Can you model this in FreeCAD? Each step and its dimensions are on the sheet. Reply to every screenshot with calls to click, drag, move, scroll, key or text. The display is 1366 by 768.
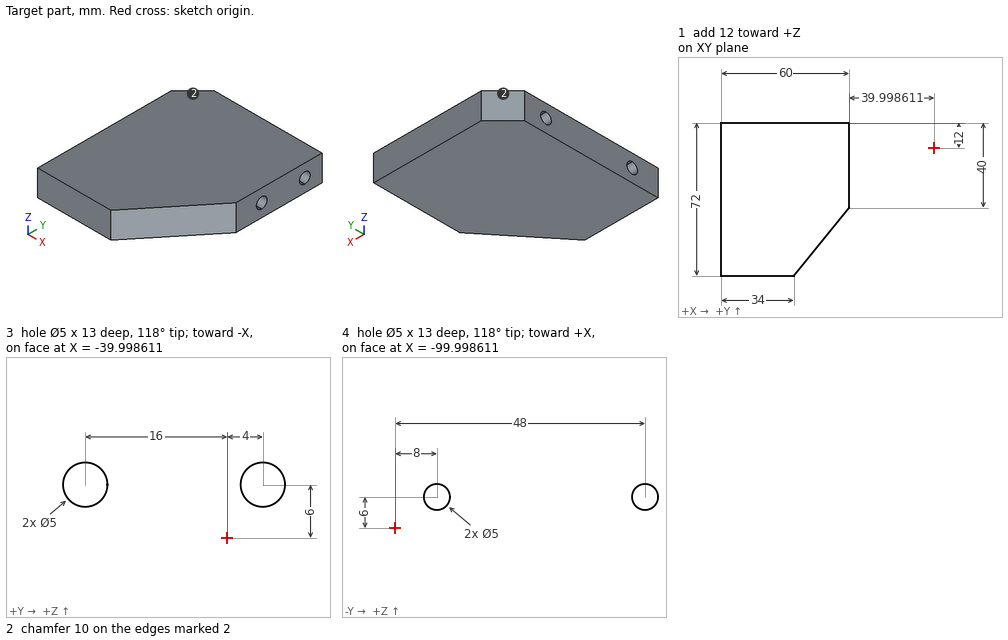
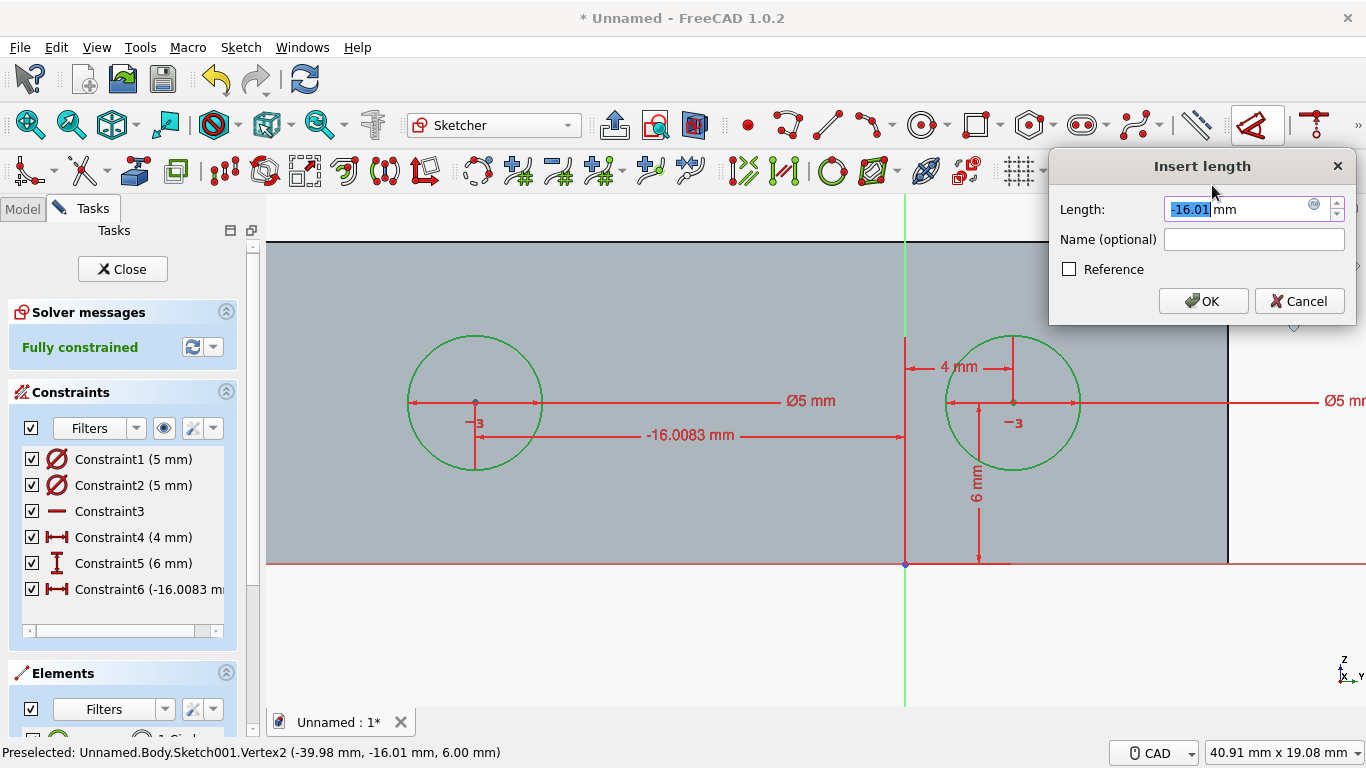
text(-16)
key(Return)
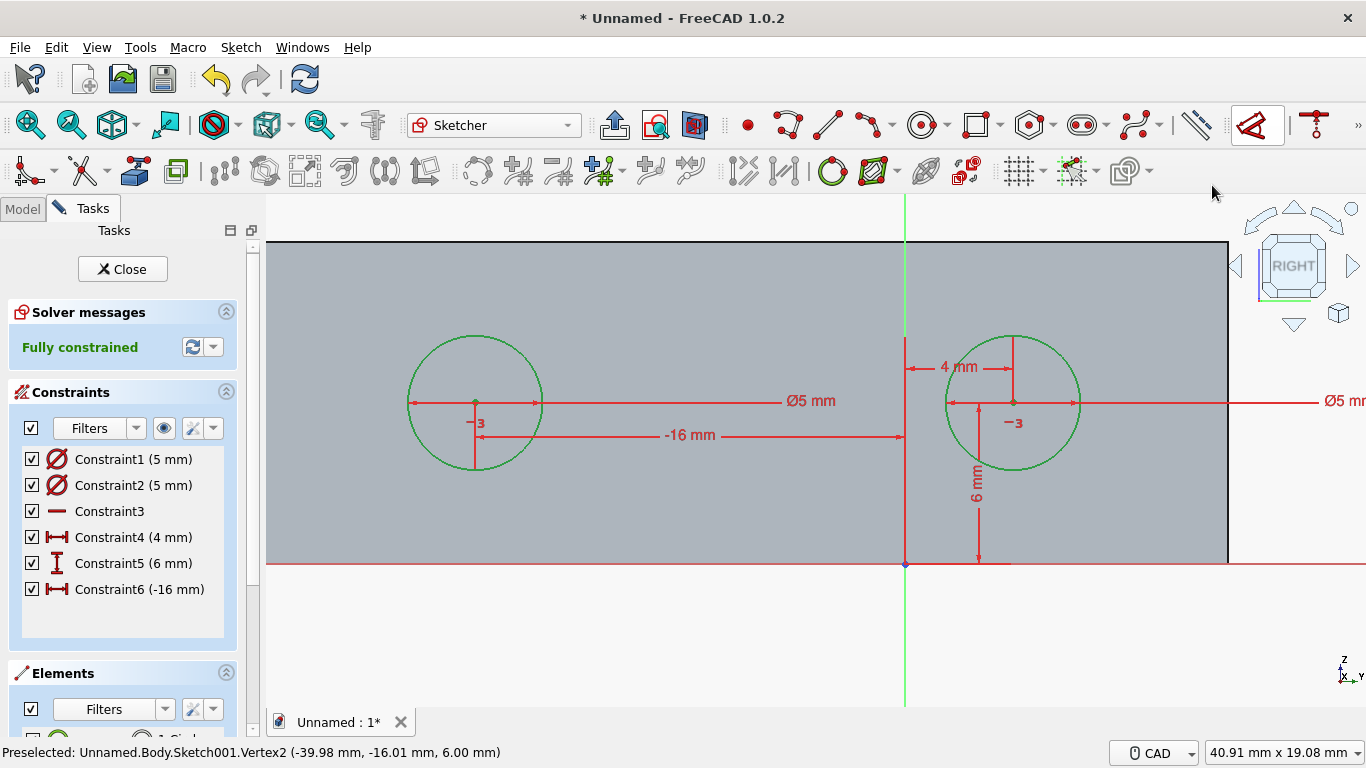
click(123, 269)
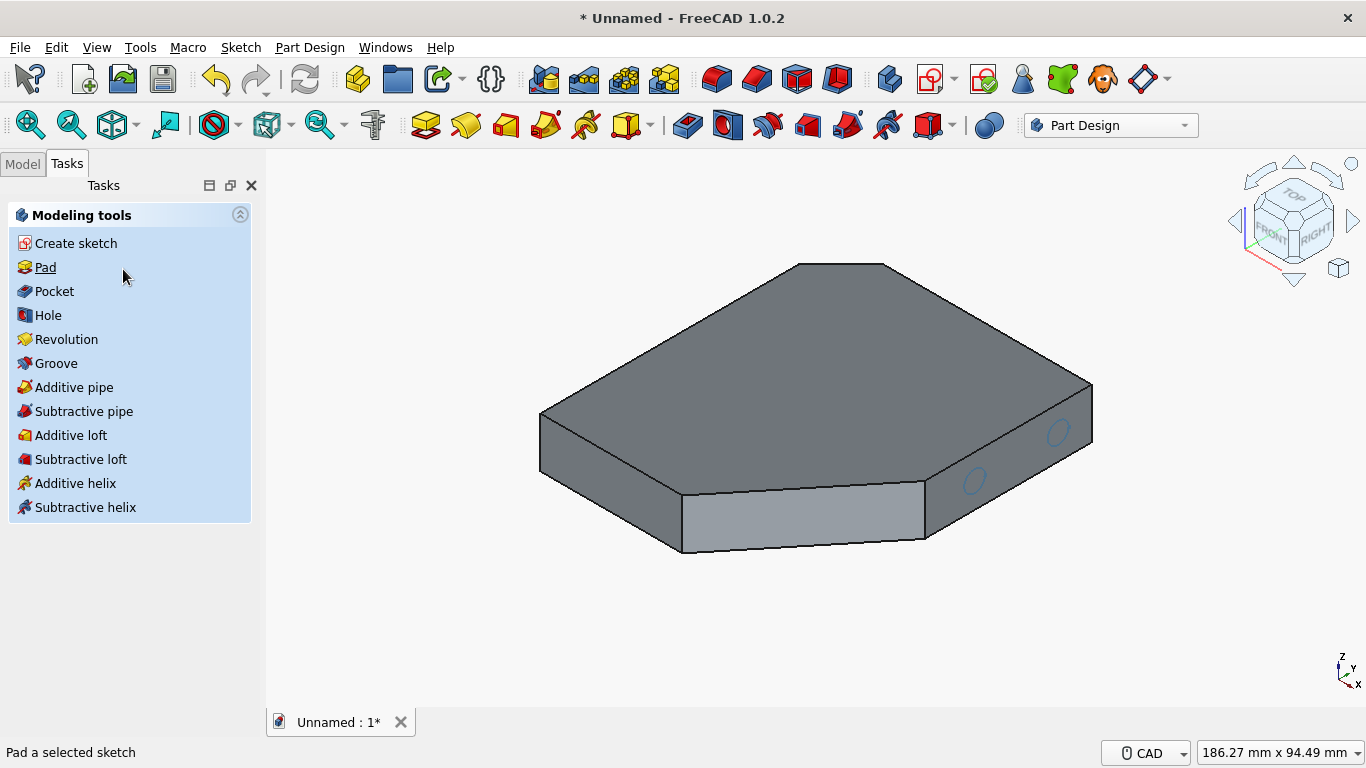
click(728, 126)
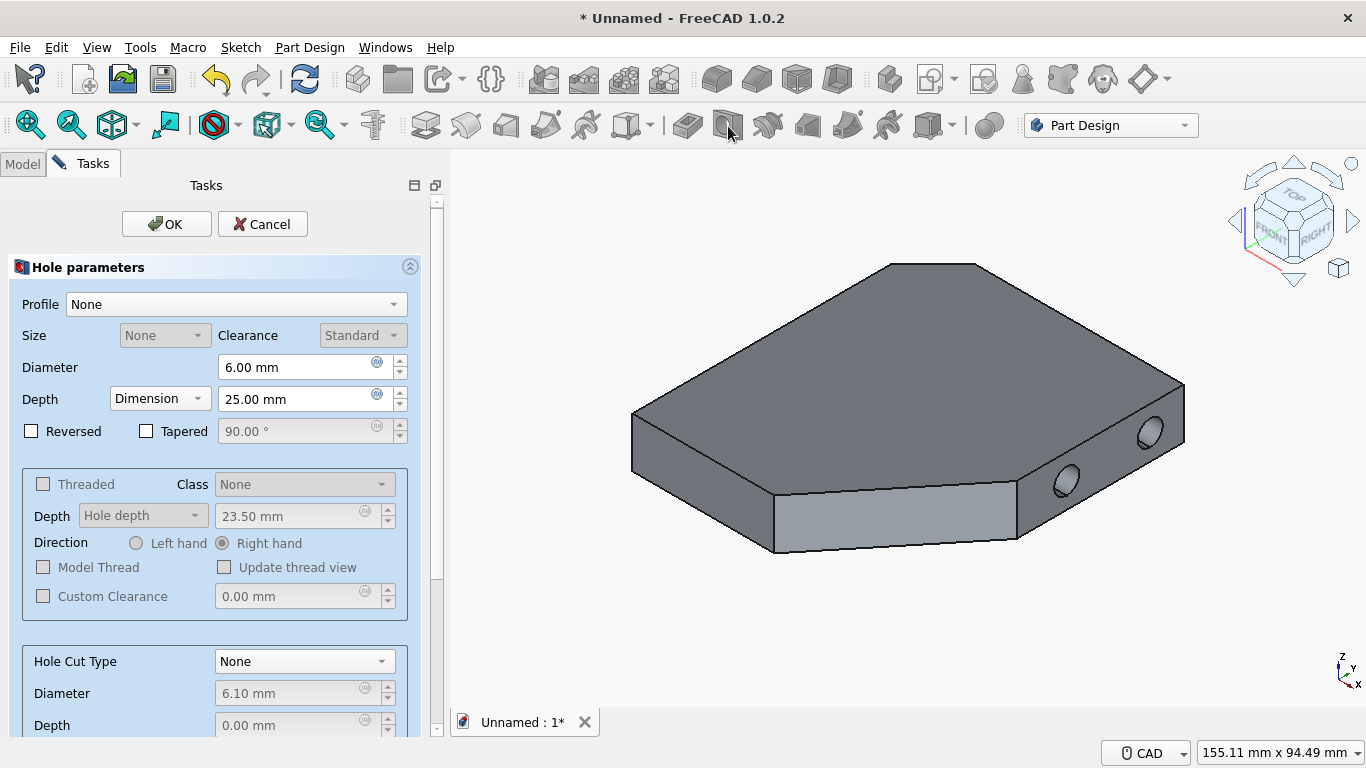
triple_click(305, 367)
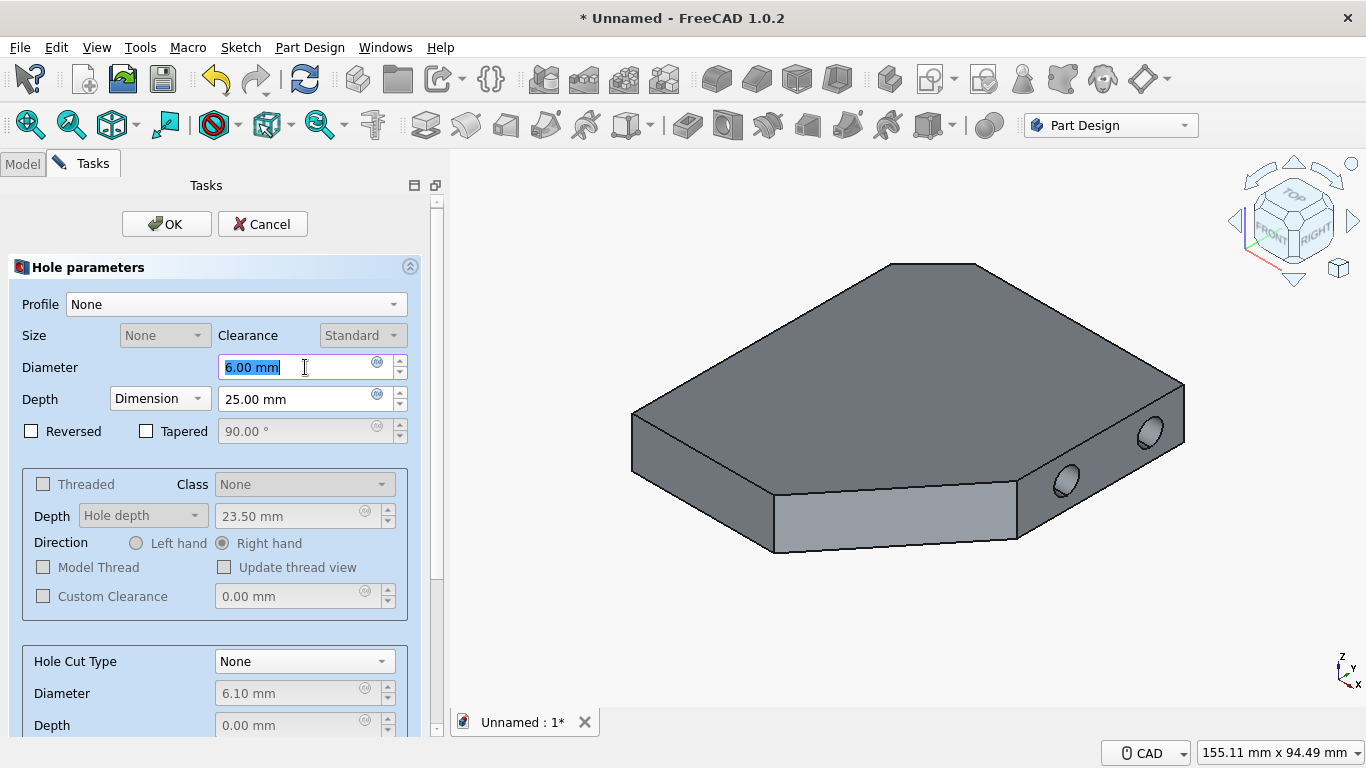
text(5)
key(Tab)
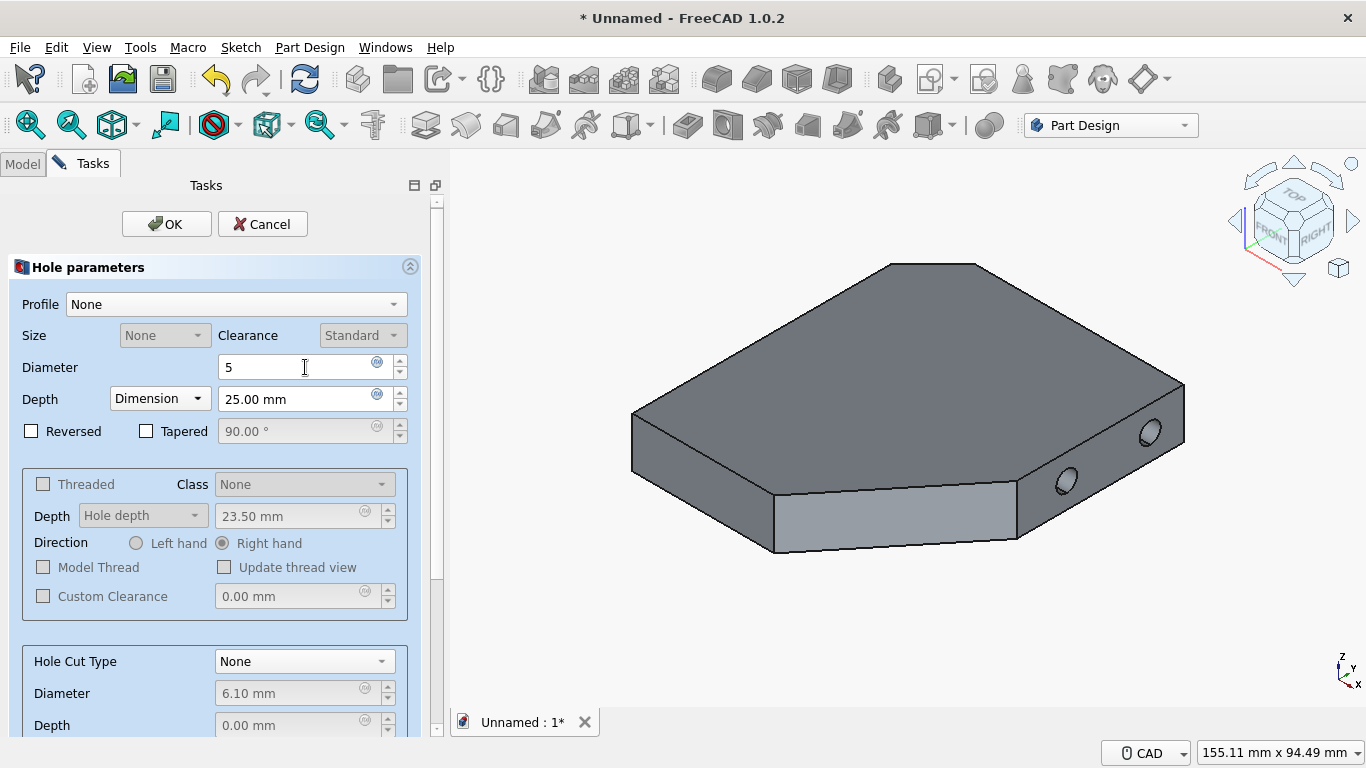
triple_click(305, 399)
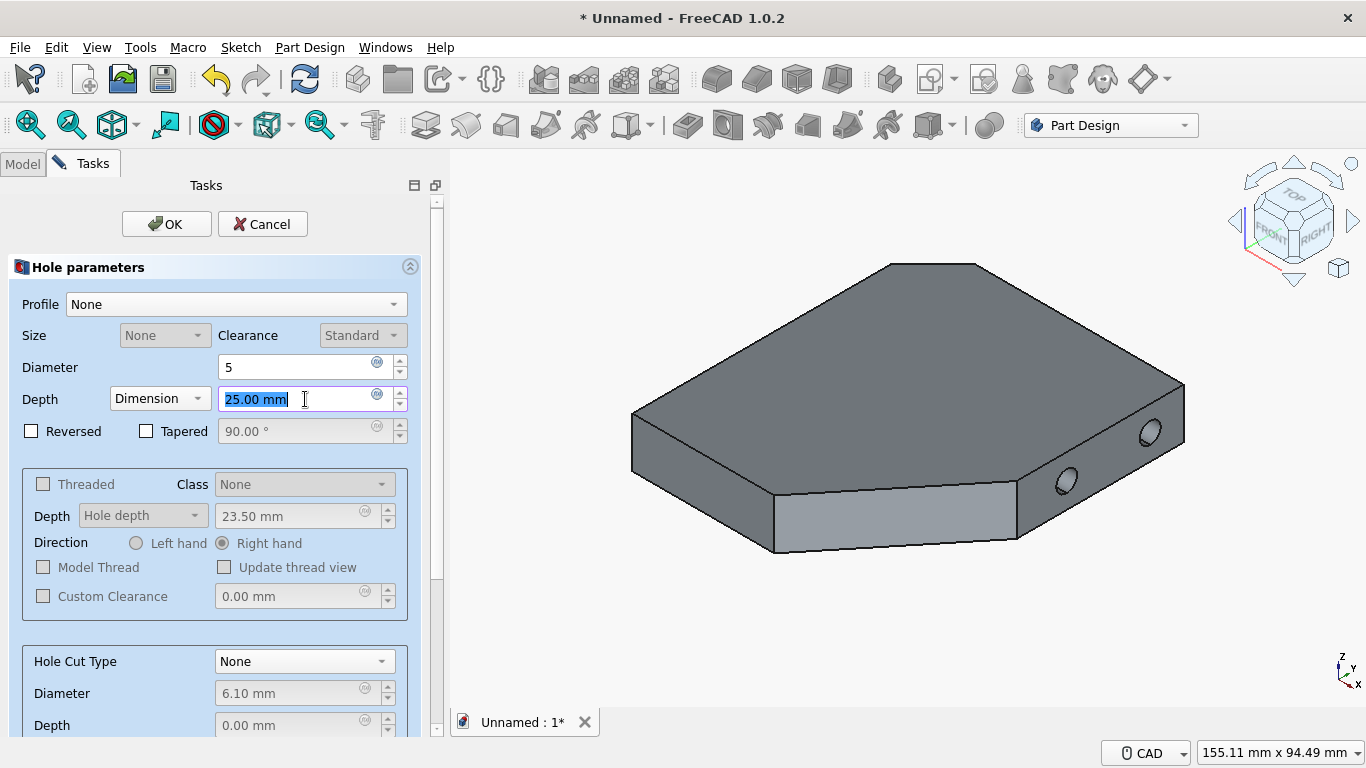
text(13)
key(Tab)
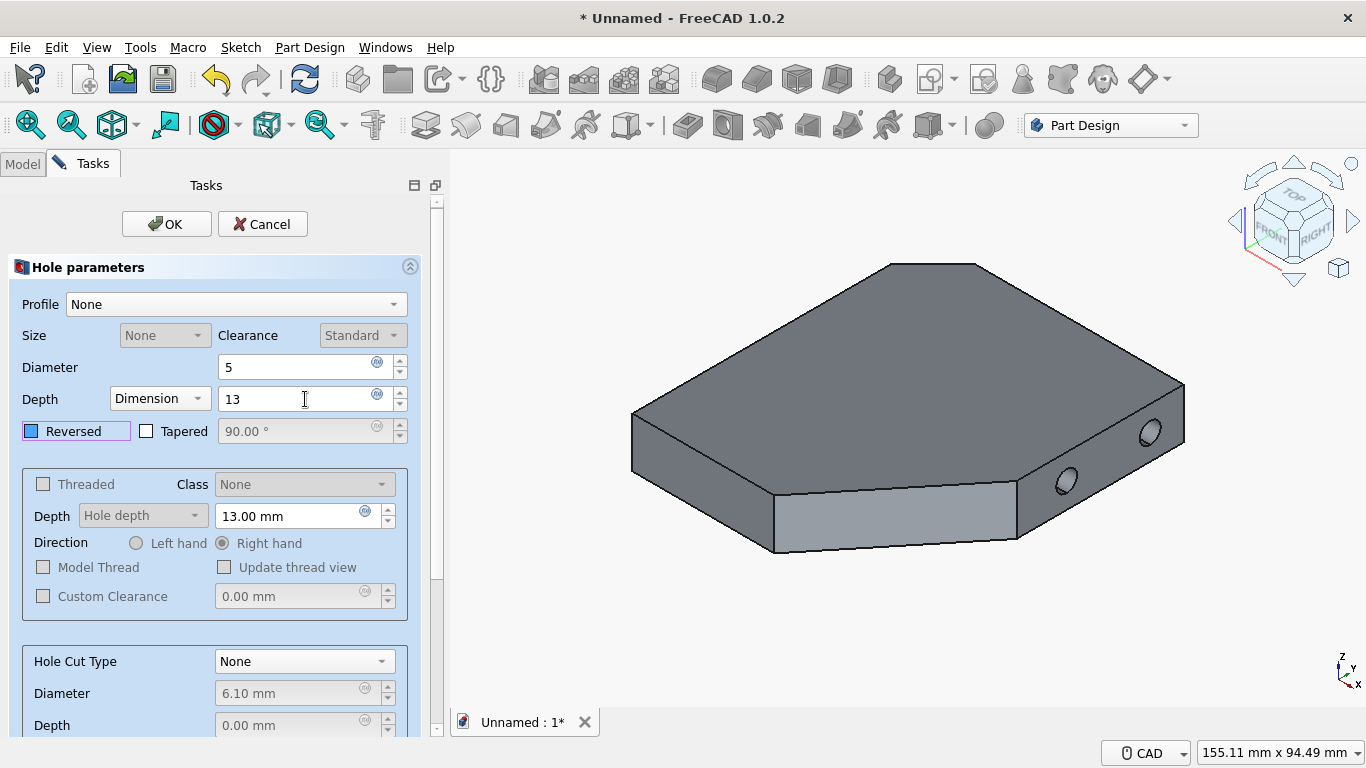
click(167, 224)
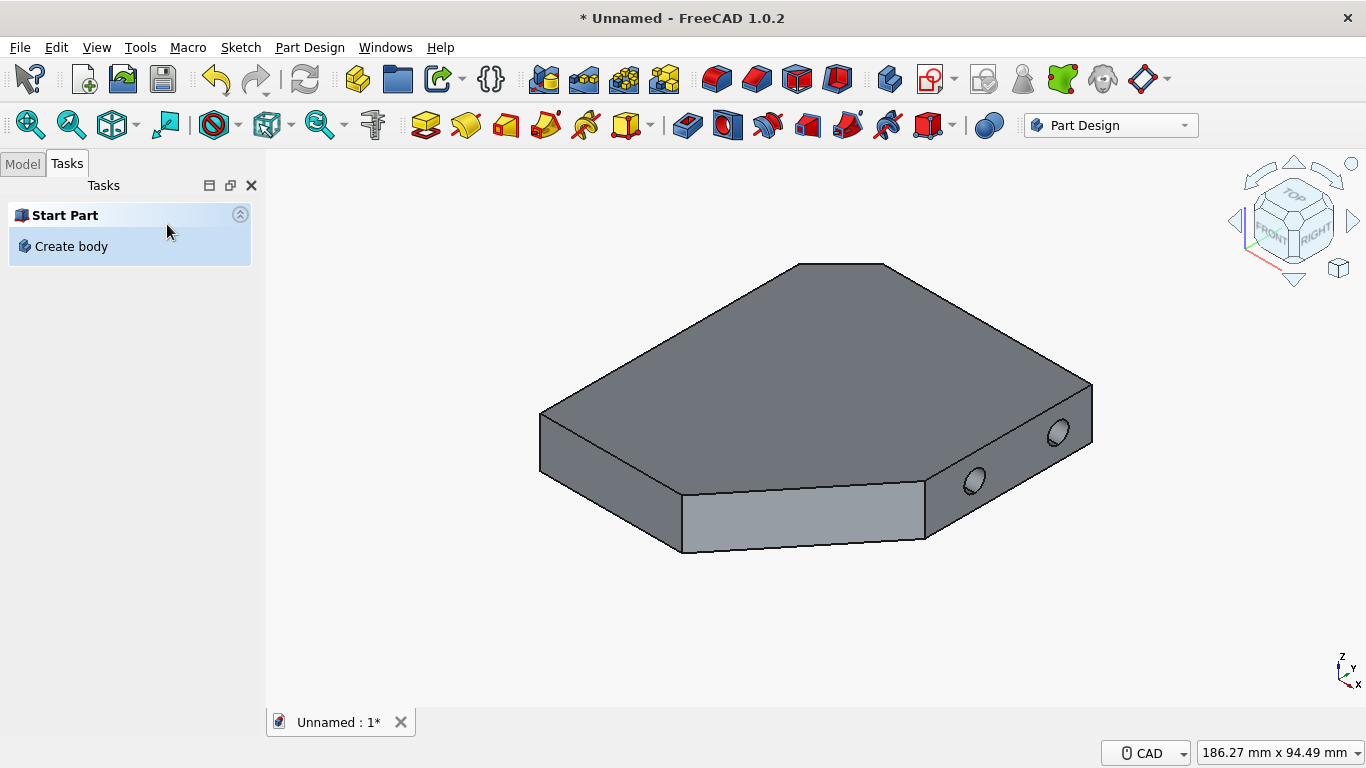
key(6)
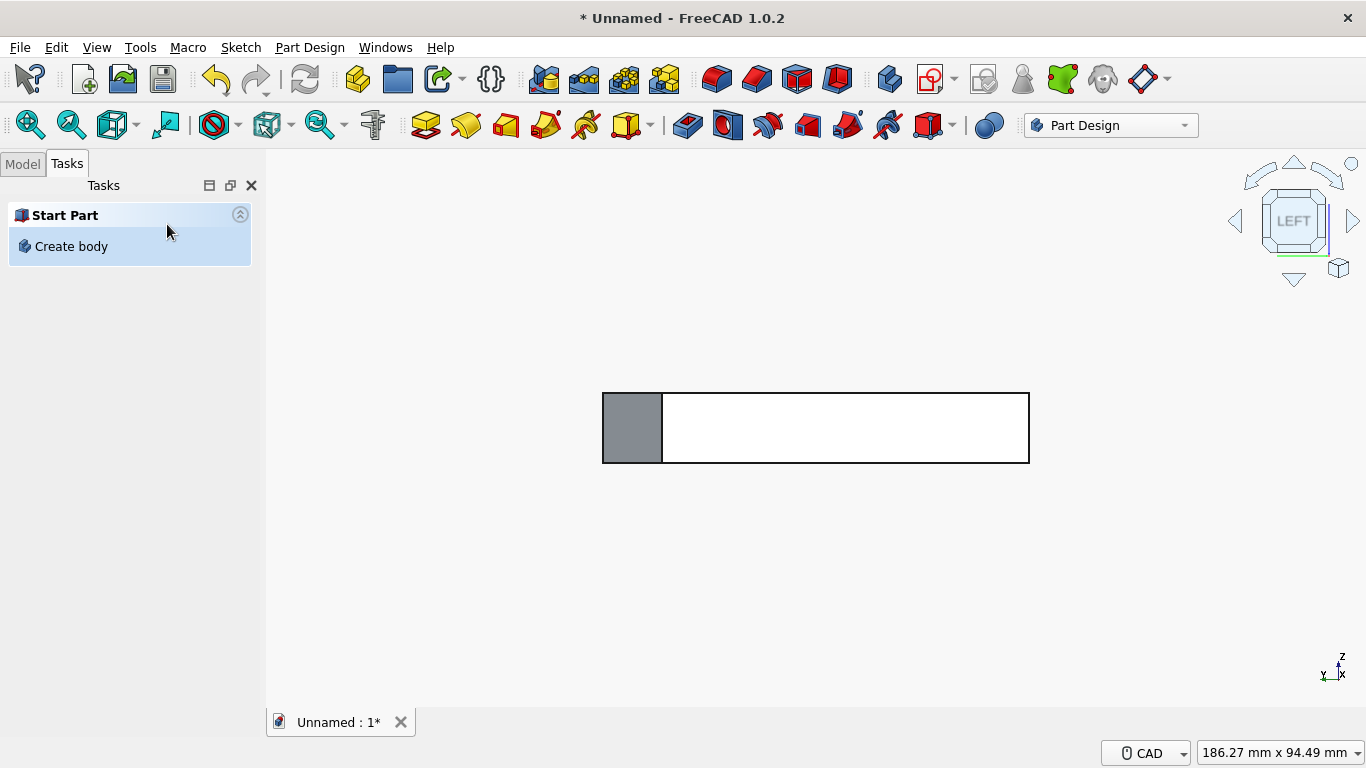
click(32, 126)